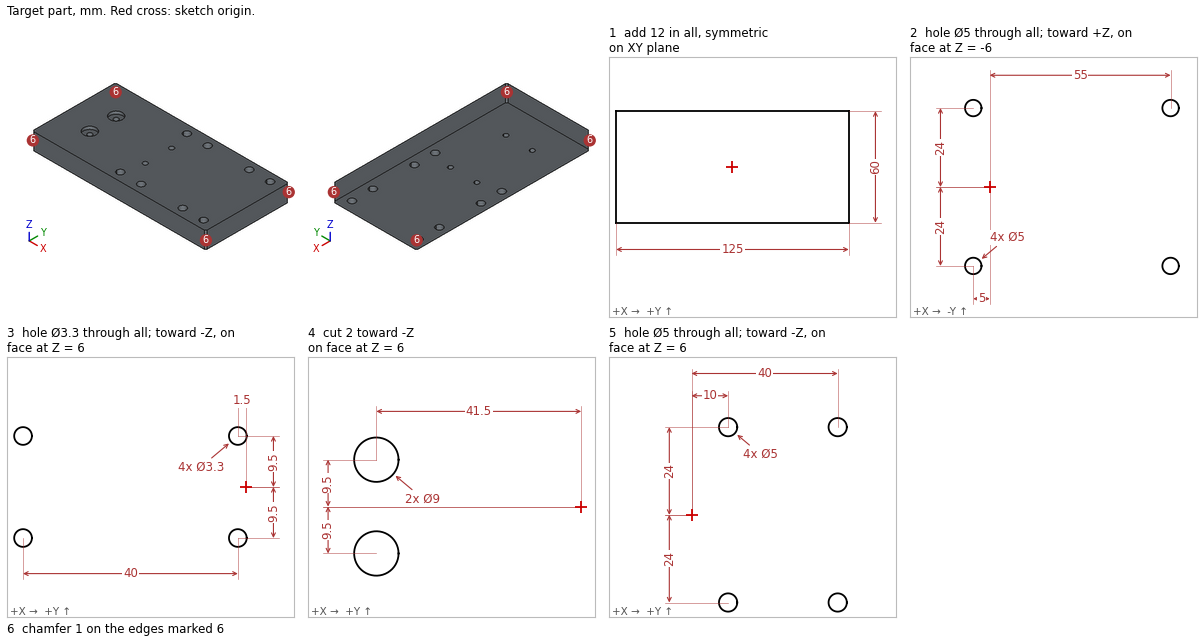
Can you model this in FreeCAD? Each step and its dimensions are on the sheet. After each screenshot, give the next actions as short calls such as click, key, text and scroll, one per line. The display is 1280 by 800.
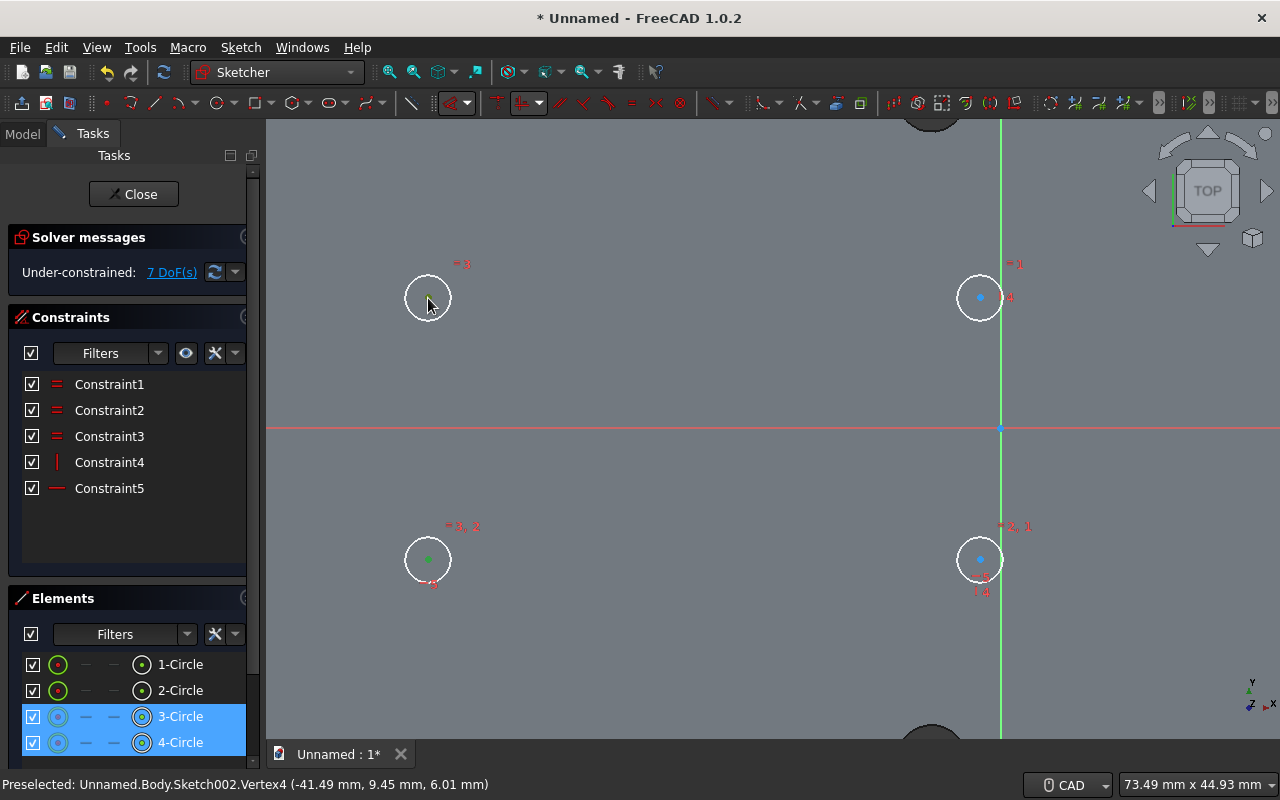
key(v)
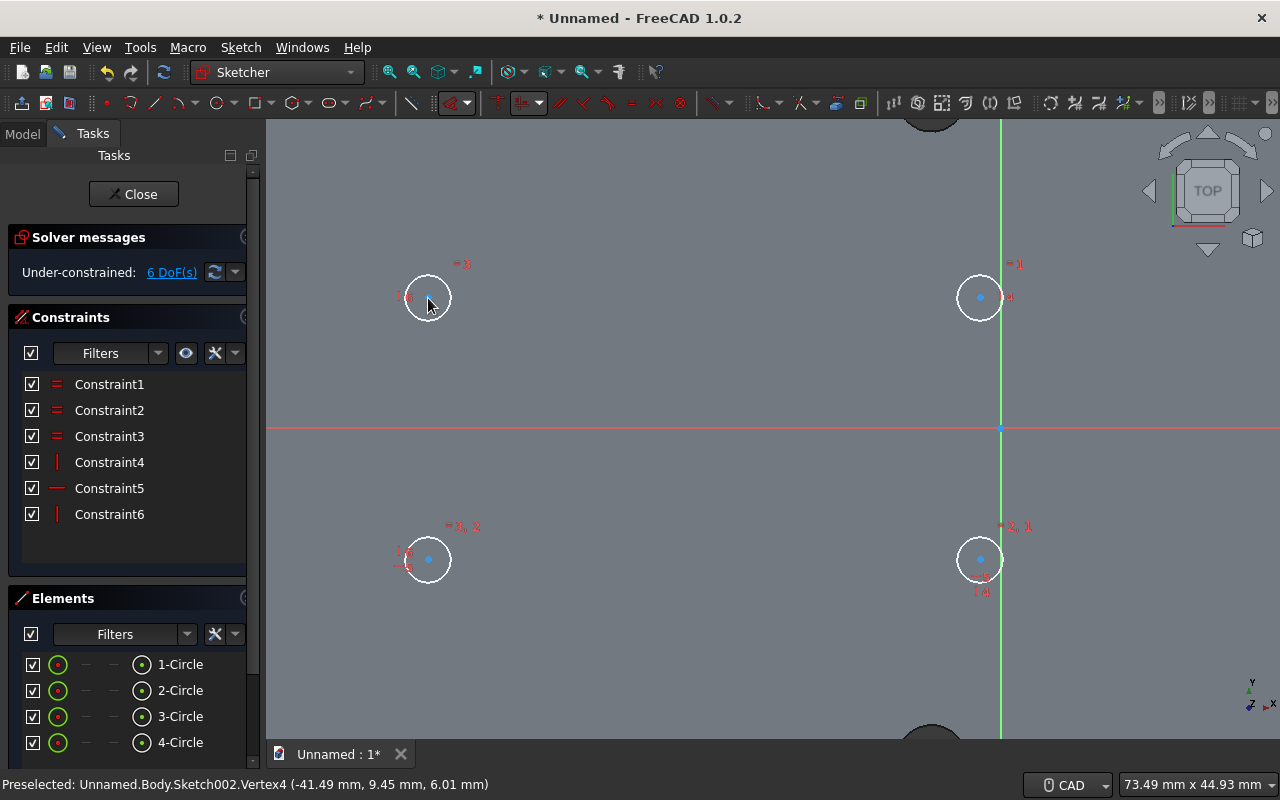
click(980, 298)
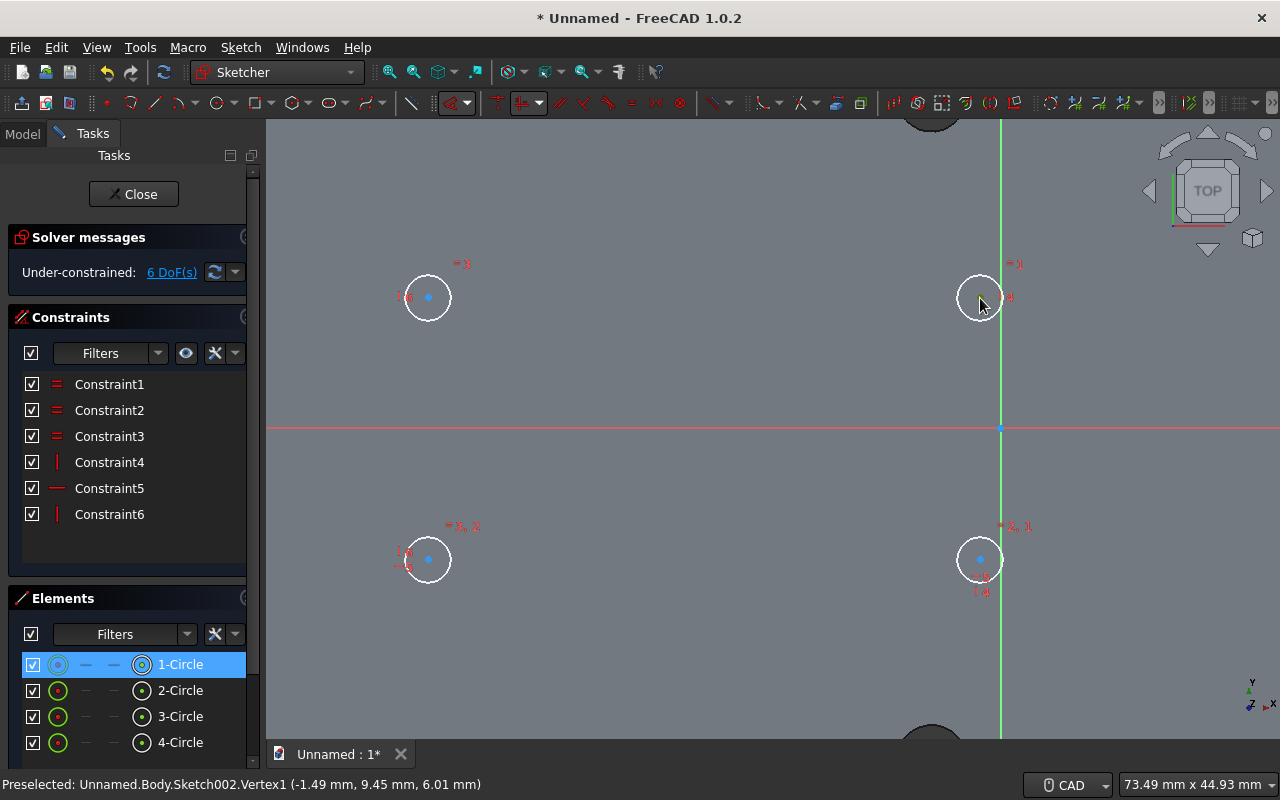
click(428, 298)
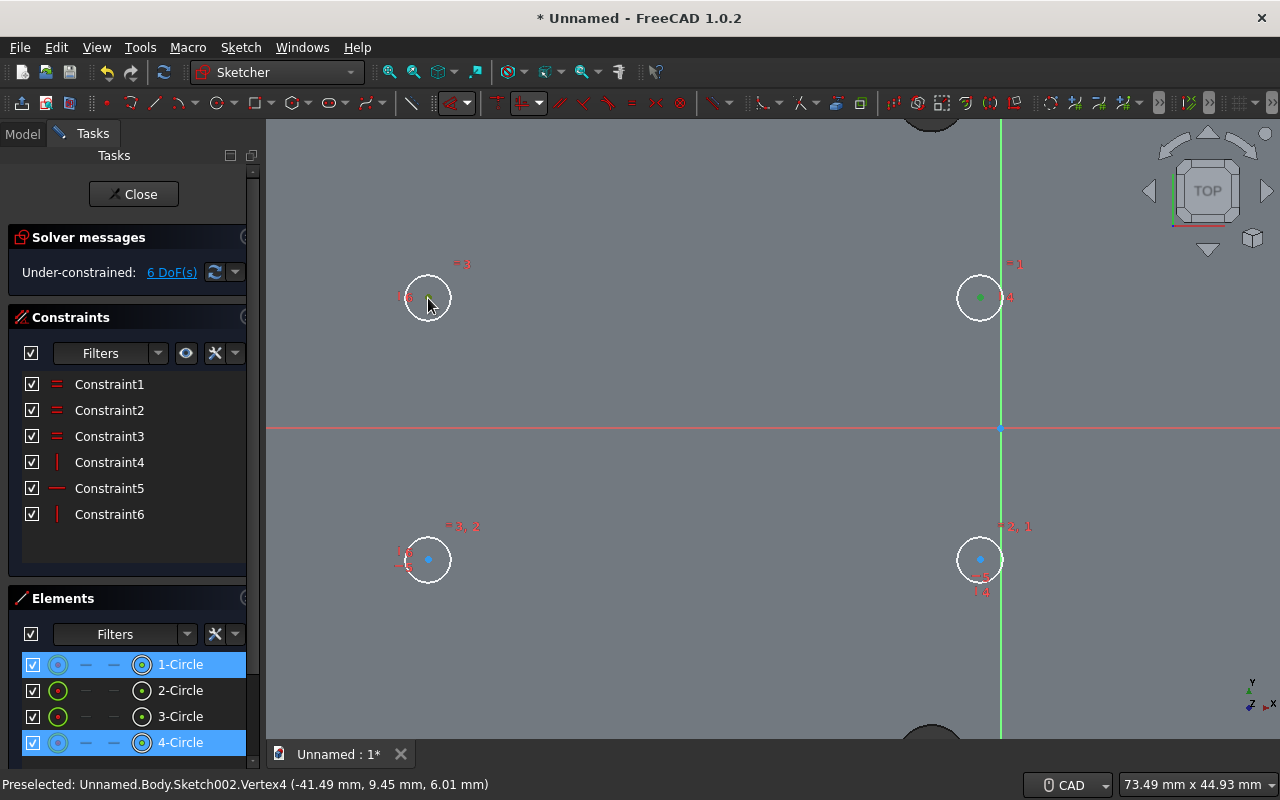
click(542, 104)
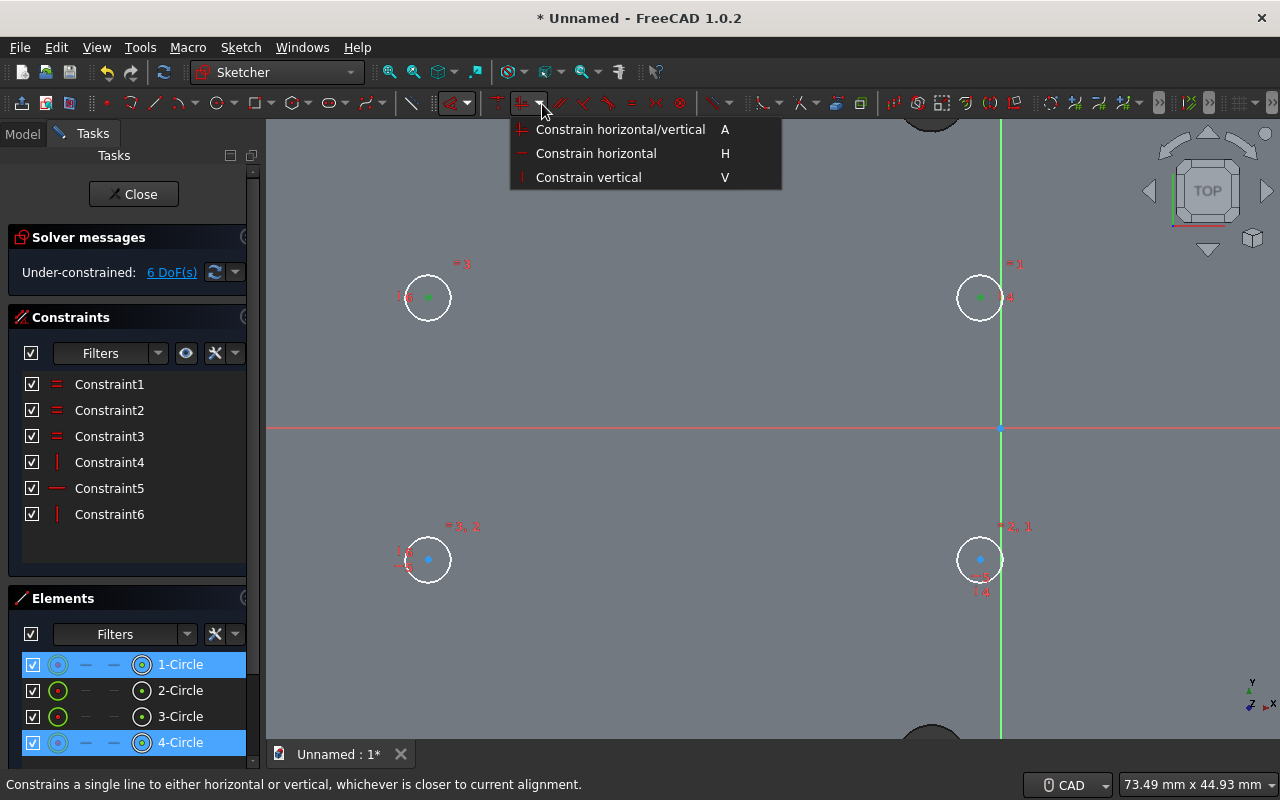
click(646, 153)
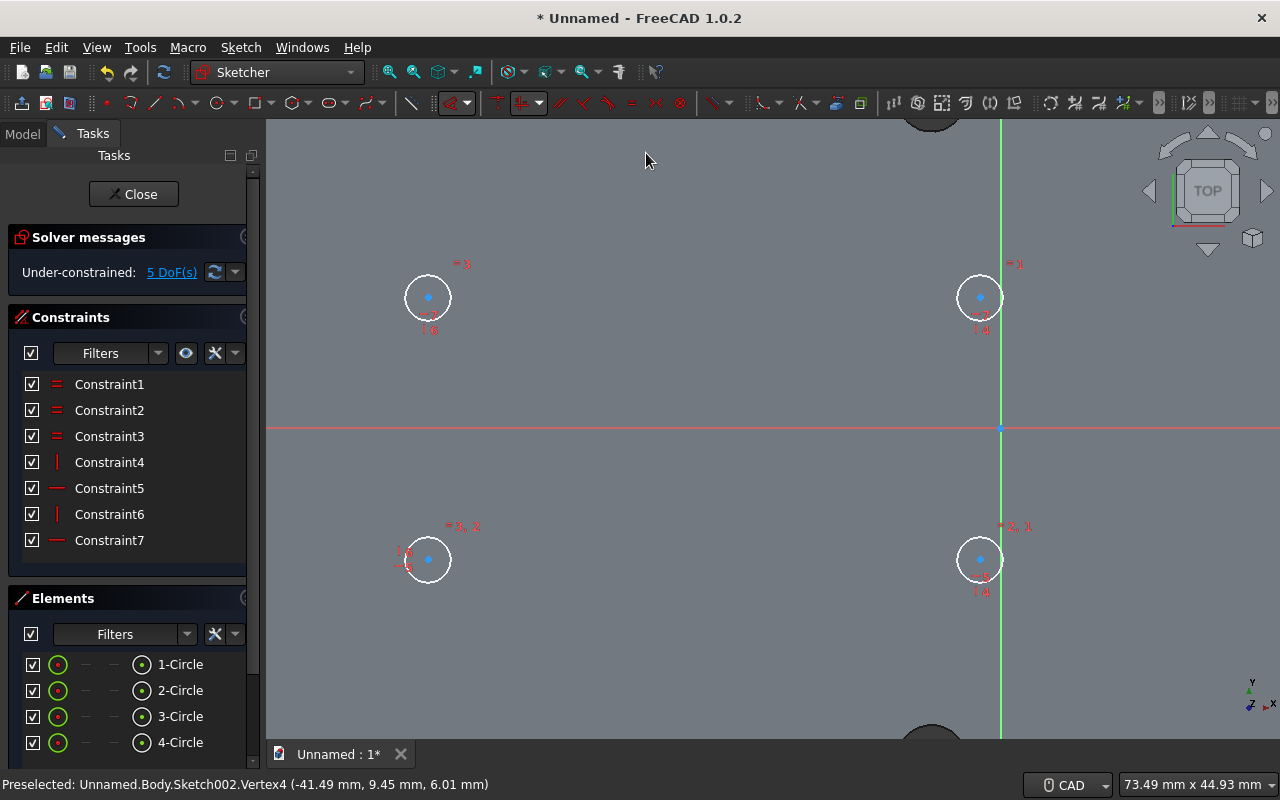
click(964, 282)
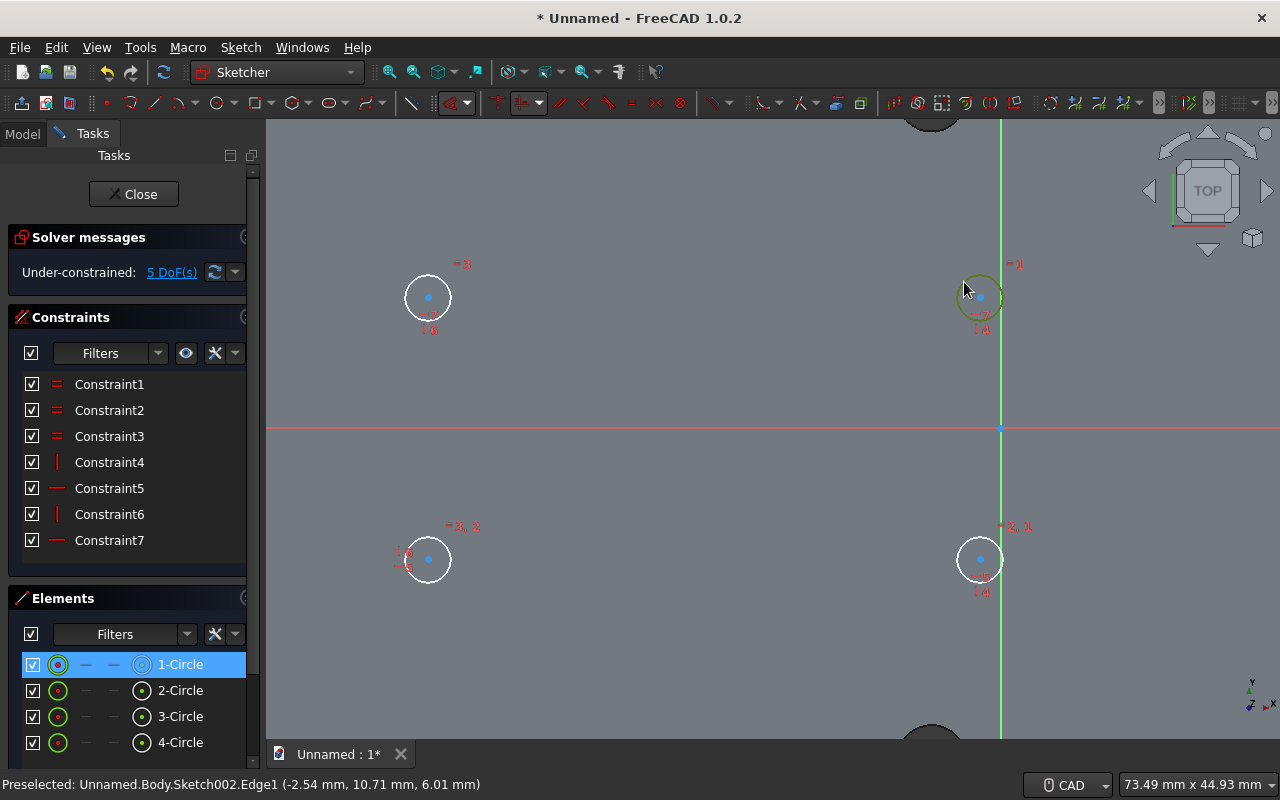
key(k)
key(o)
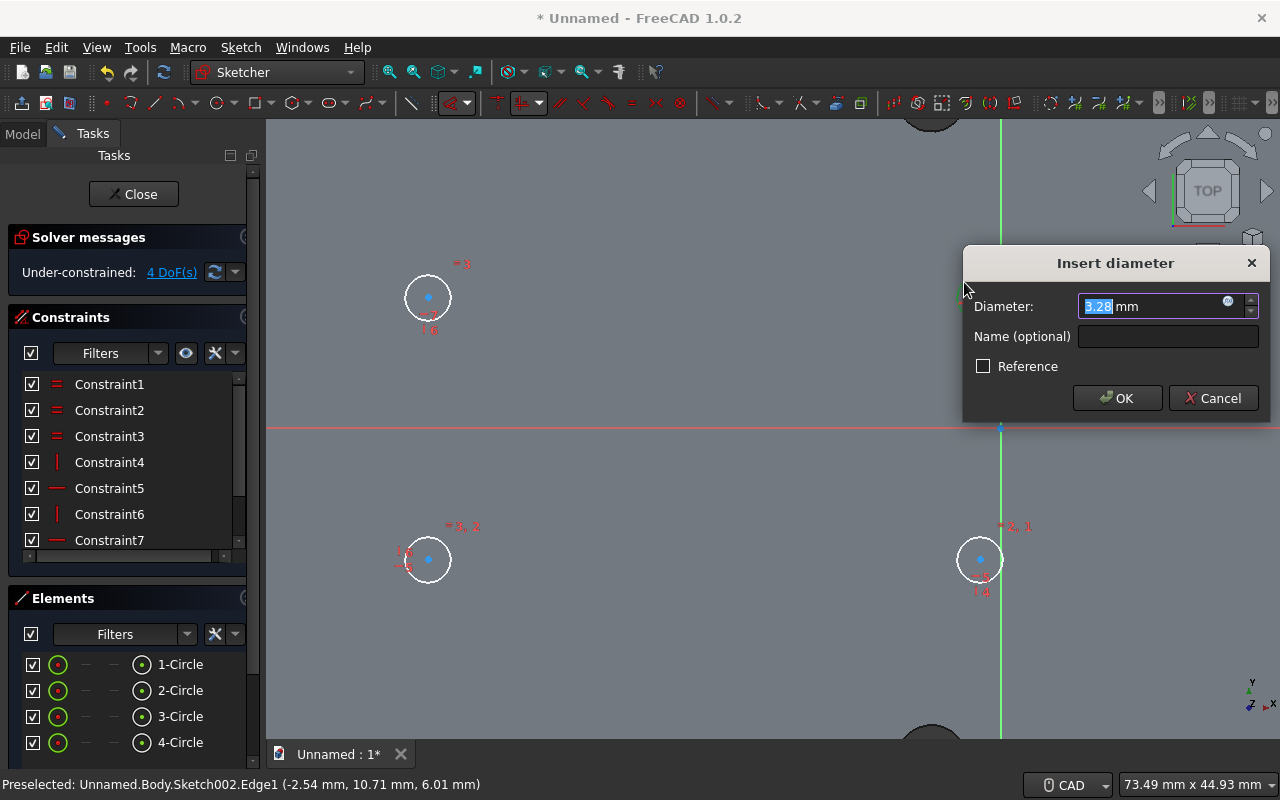
text(3.3)
key(Return)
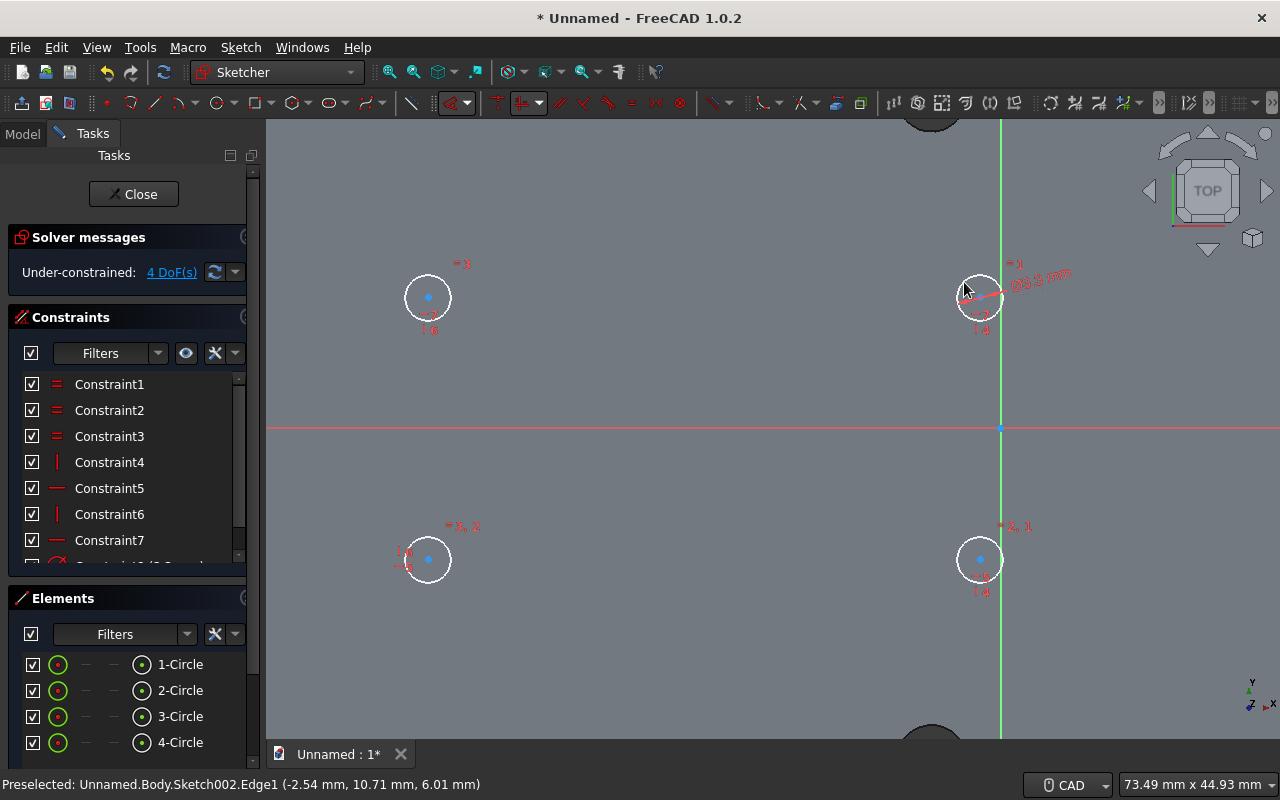
scroll(980, 298, up, 4)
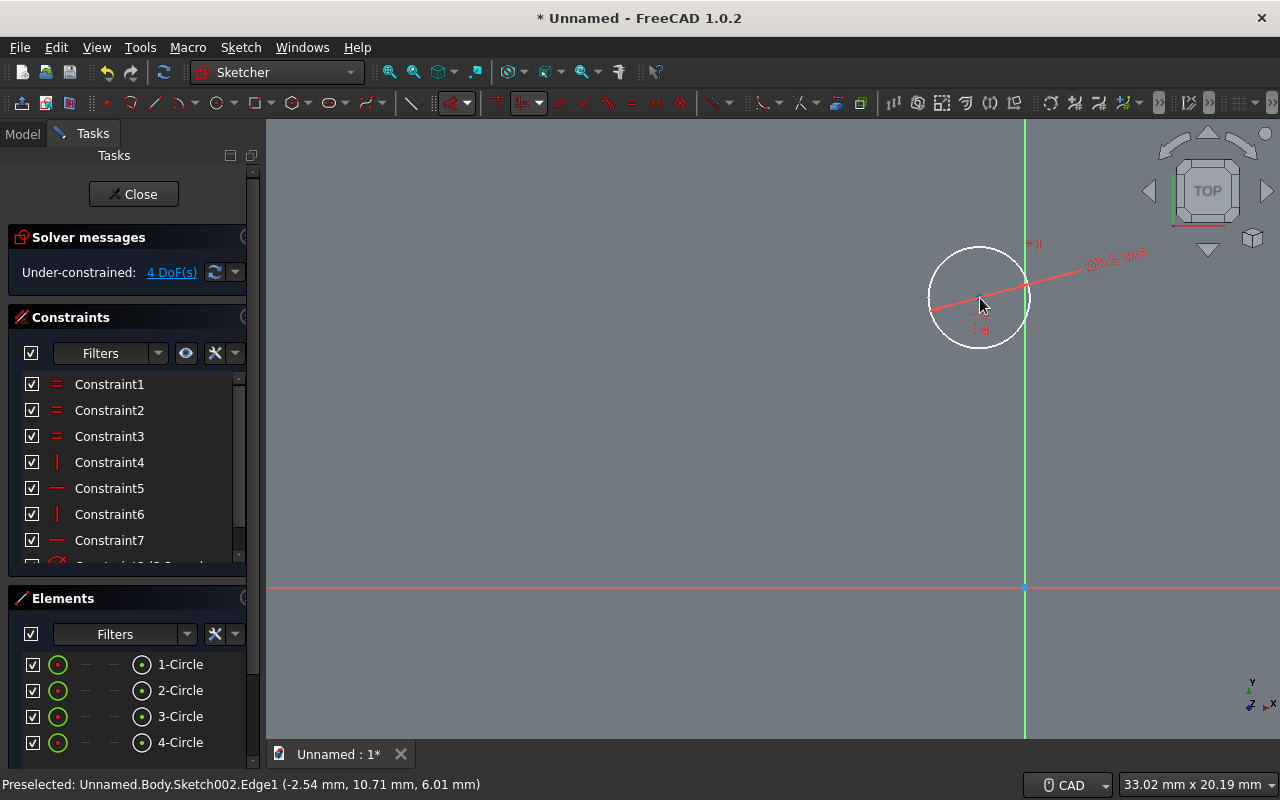
click(979, 298)